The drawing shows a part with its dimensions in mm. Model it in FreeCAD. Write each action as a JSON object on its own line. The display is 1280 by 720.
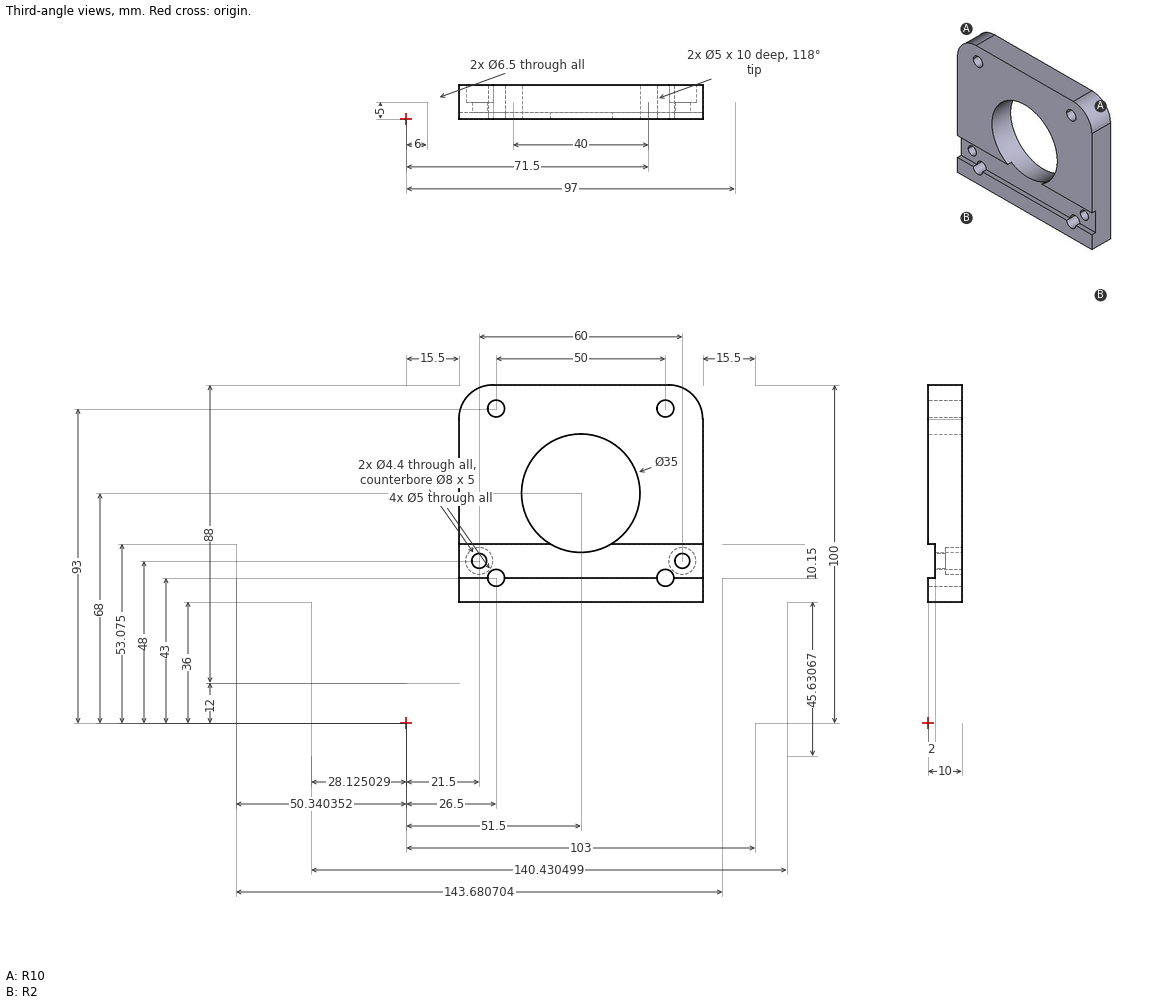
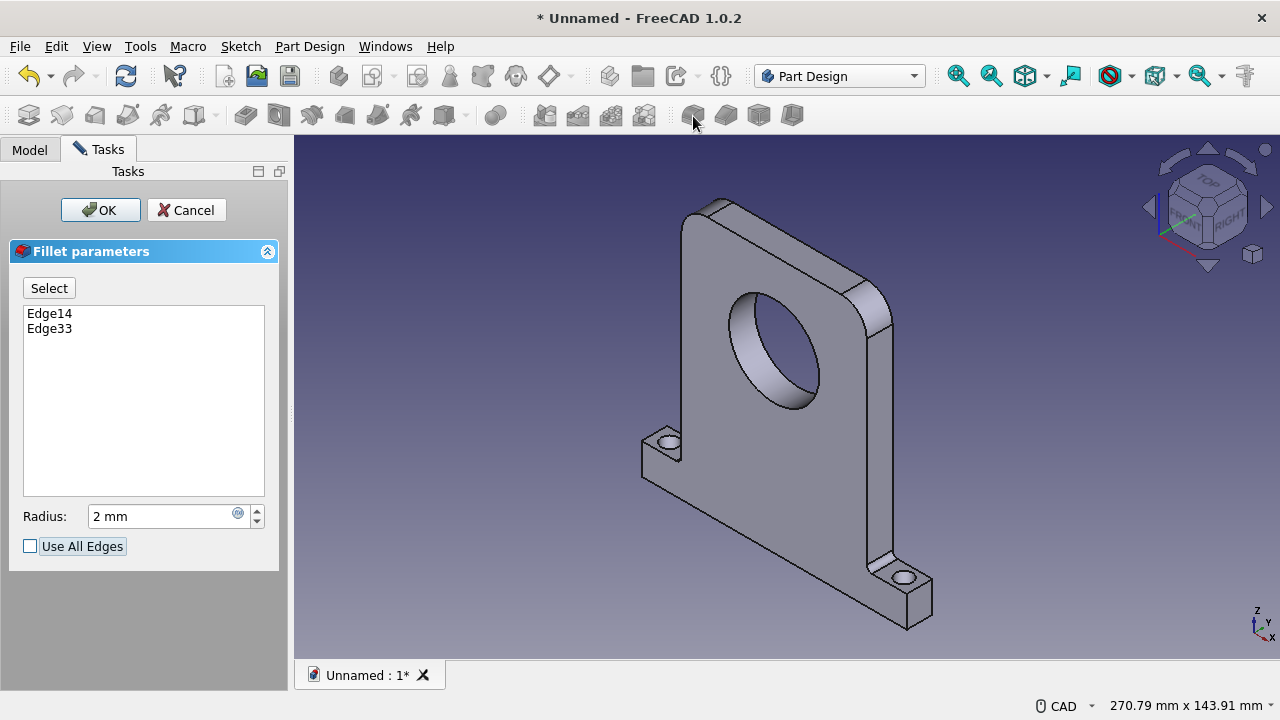
{"action": "left_click", "coordinate": [101, 210]}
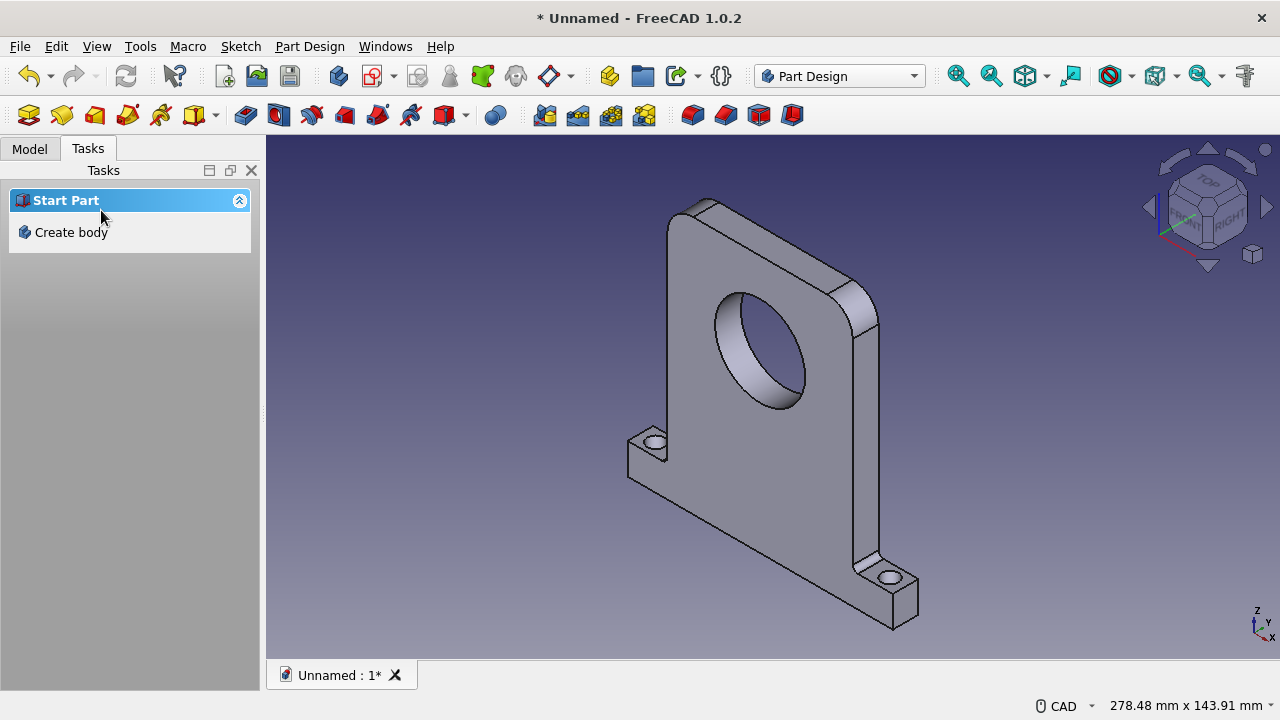
{"action": "key", "text": "4"}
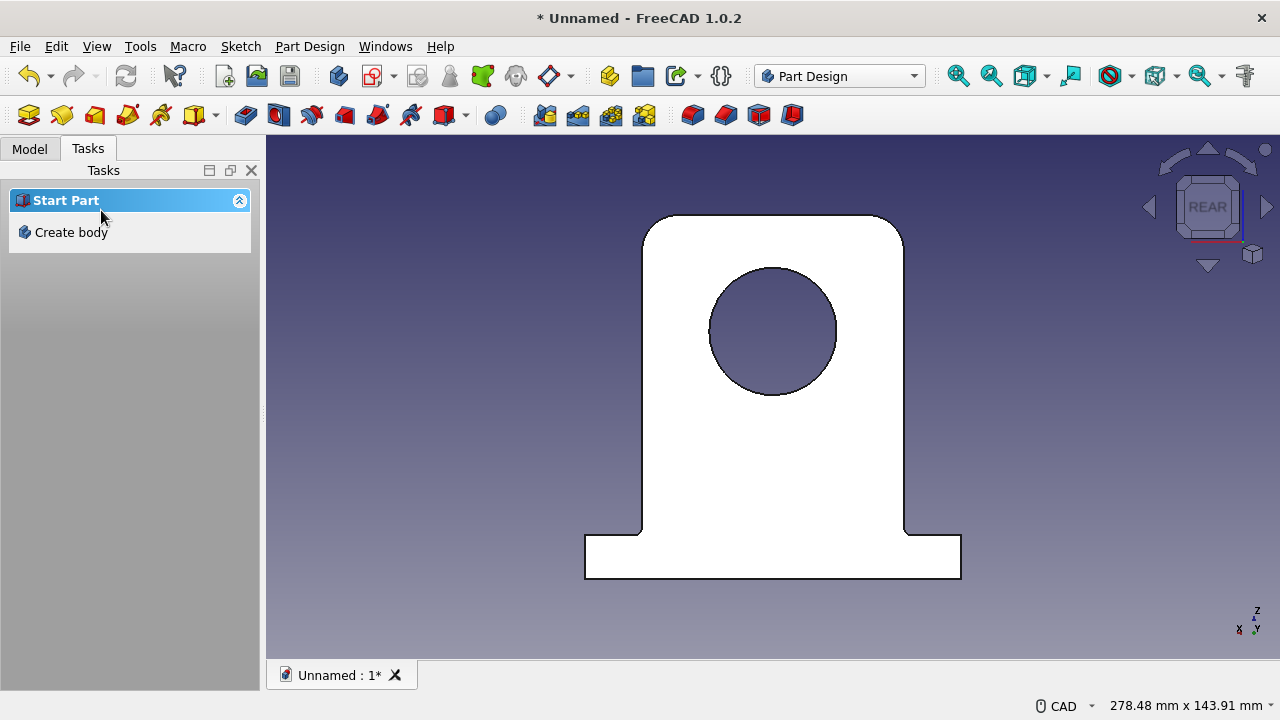
{"action": "left_click", "coordinate": [773, 500]}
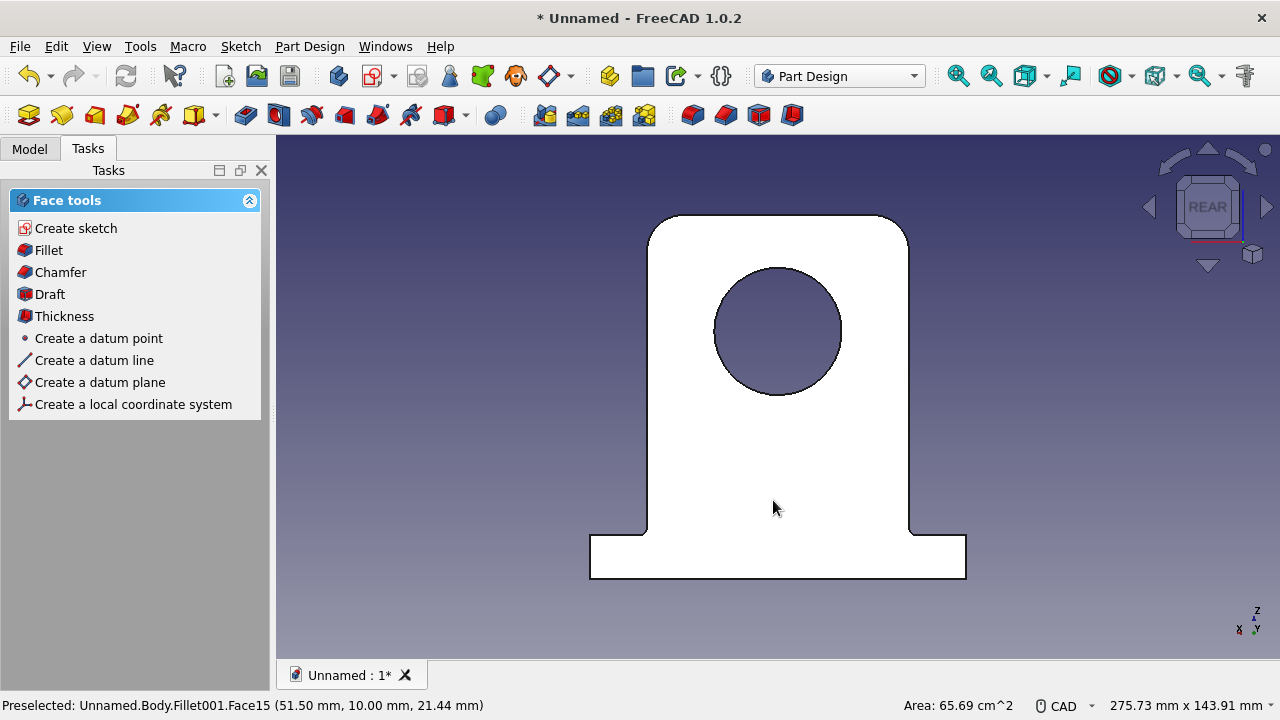
{"action": "left_click", "coordinate": [372, 76]}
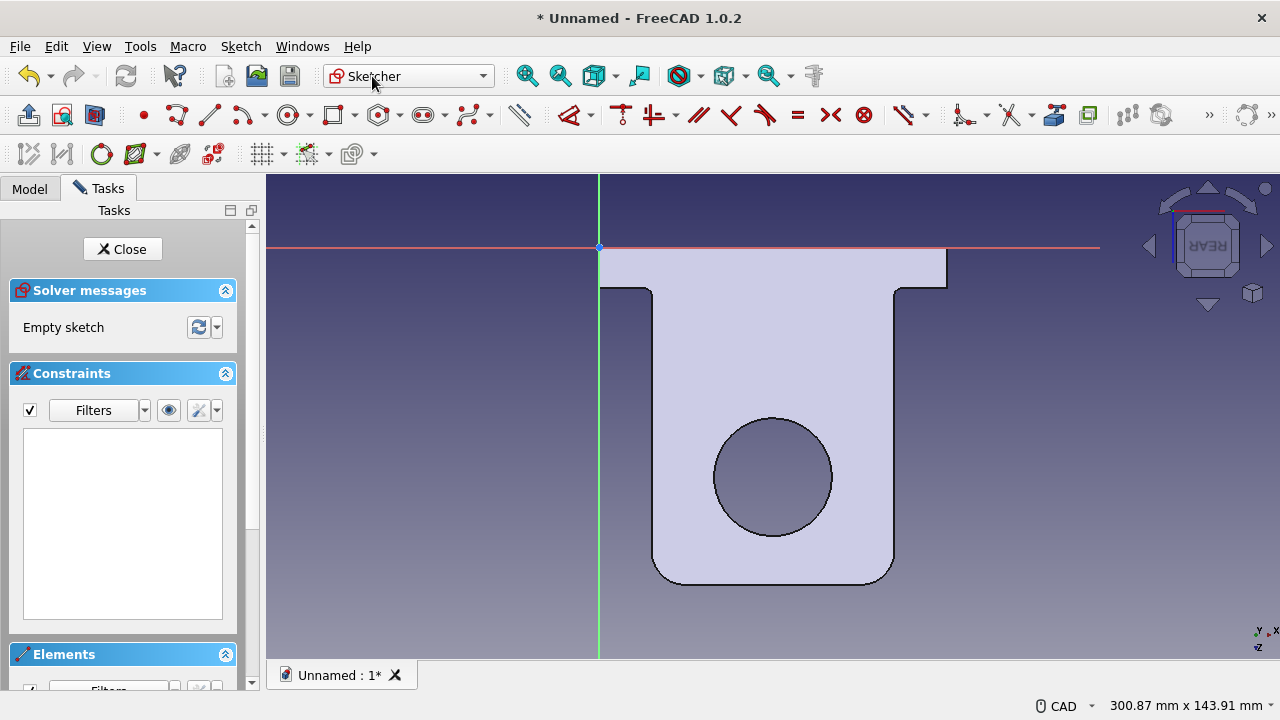
{"action": "scroll", "coordinate": [538, 631], "scroll_direction": "down", "scroll_amount": 1}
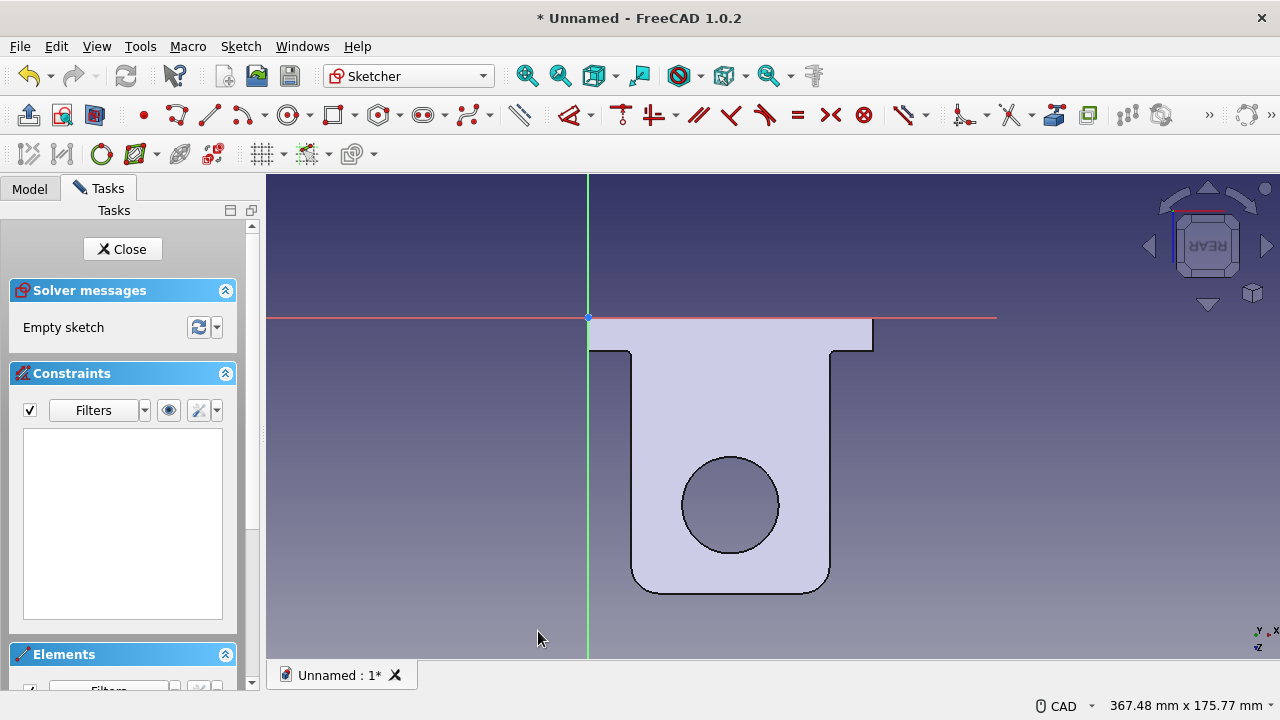
{"action": "scroll", "coordinate": [704, 227], "scroll_direction": "up", "scroll_amount": 2}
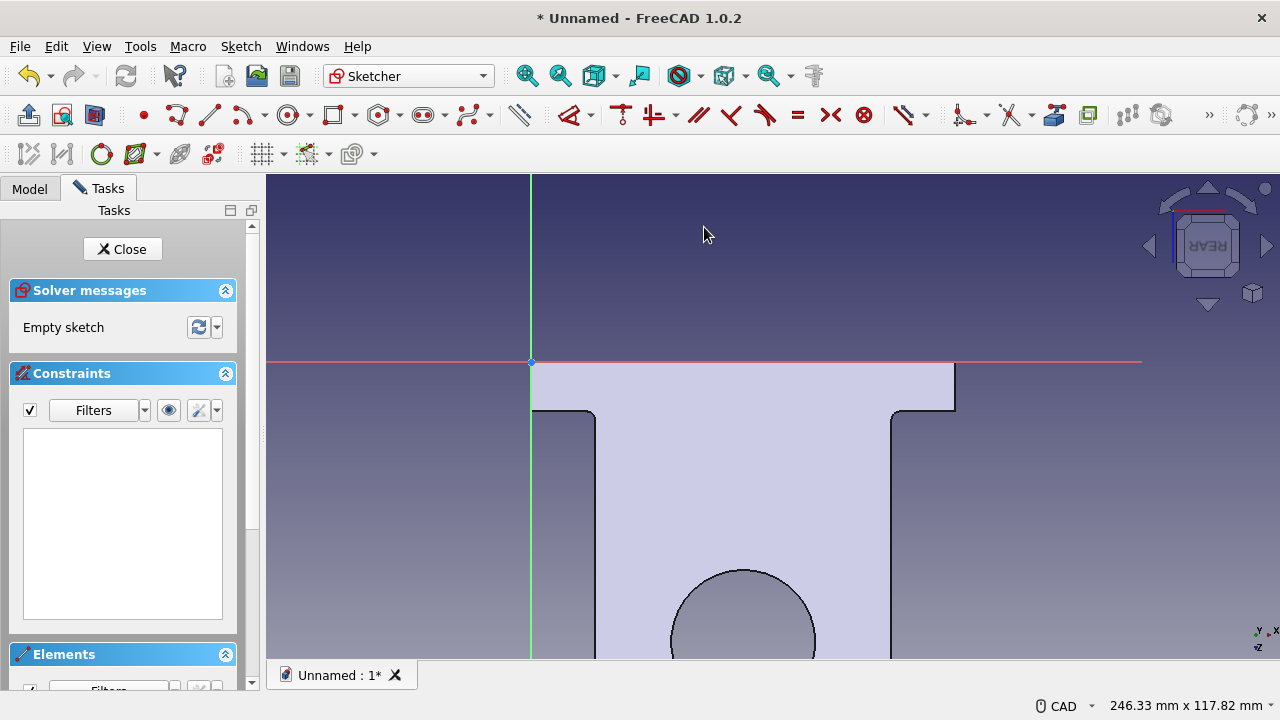
{"action": "left_click", "coordinate": [332, 116]}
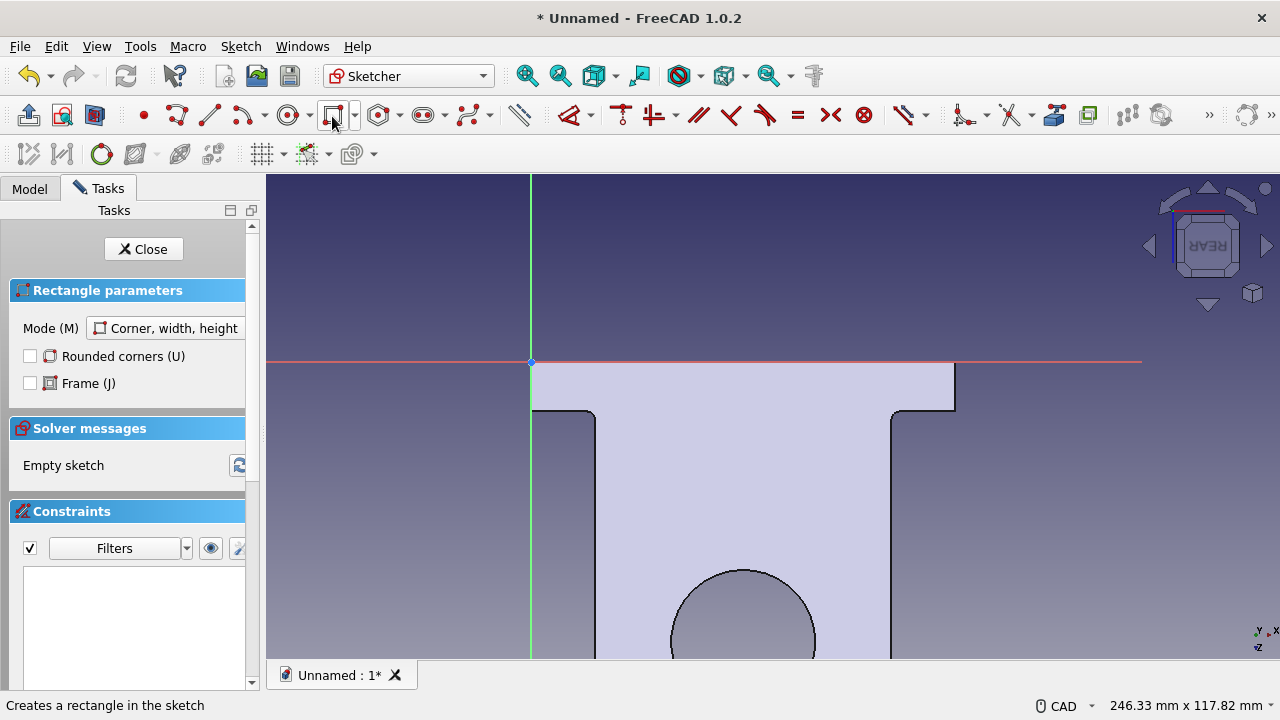
{"action": "left_click", "coordinate": [415, 322]}
{"action": "mouse_move", "coordinate": [994, 510]}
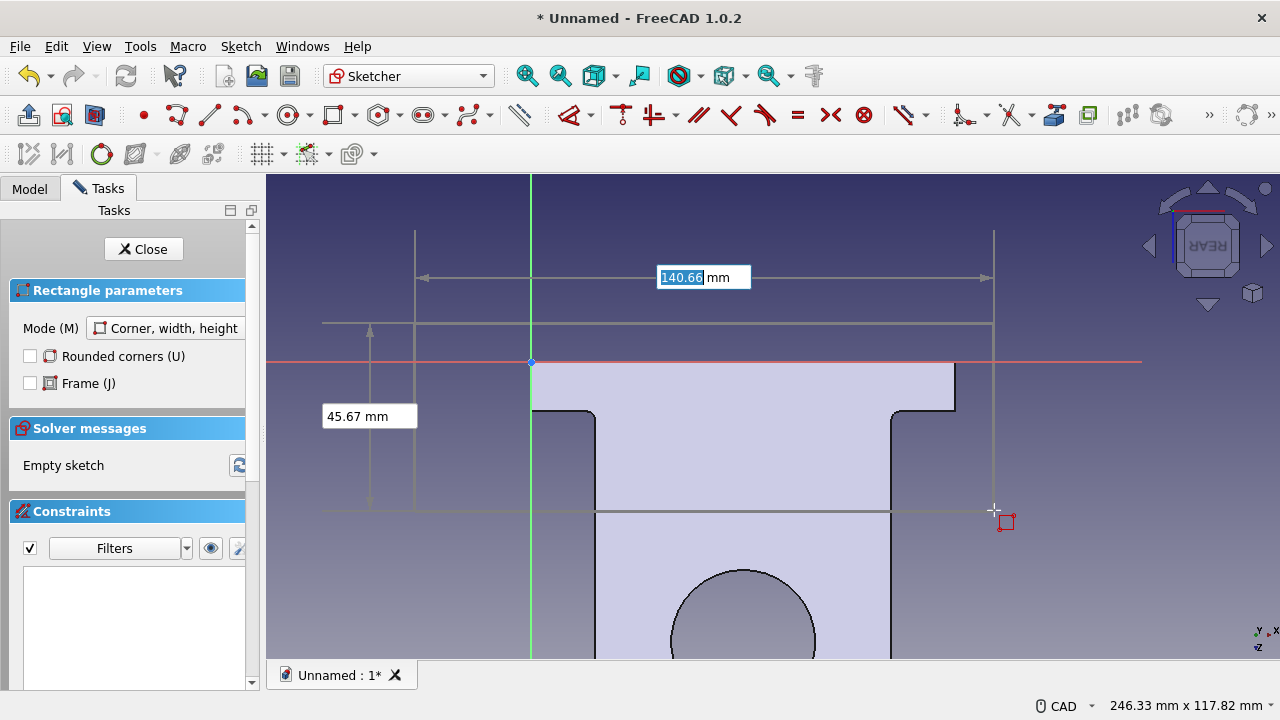
{"action": "type", "text": "140.430499"}
{"action": "key", "text": "Tab"}
{"action": "type", "text": "45.63067"}
{"action": "key", "text": "Return"}
{"action": "key", "text": "Escape"}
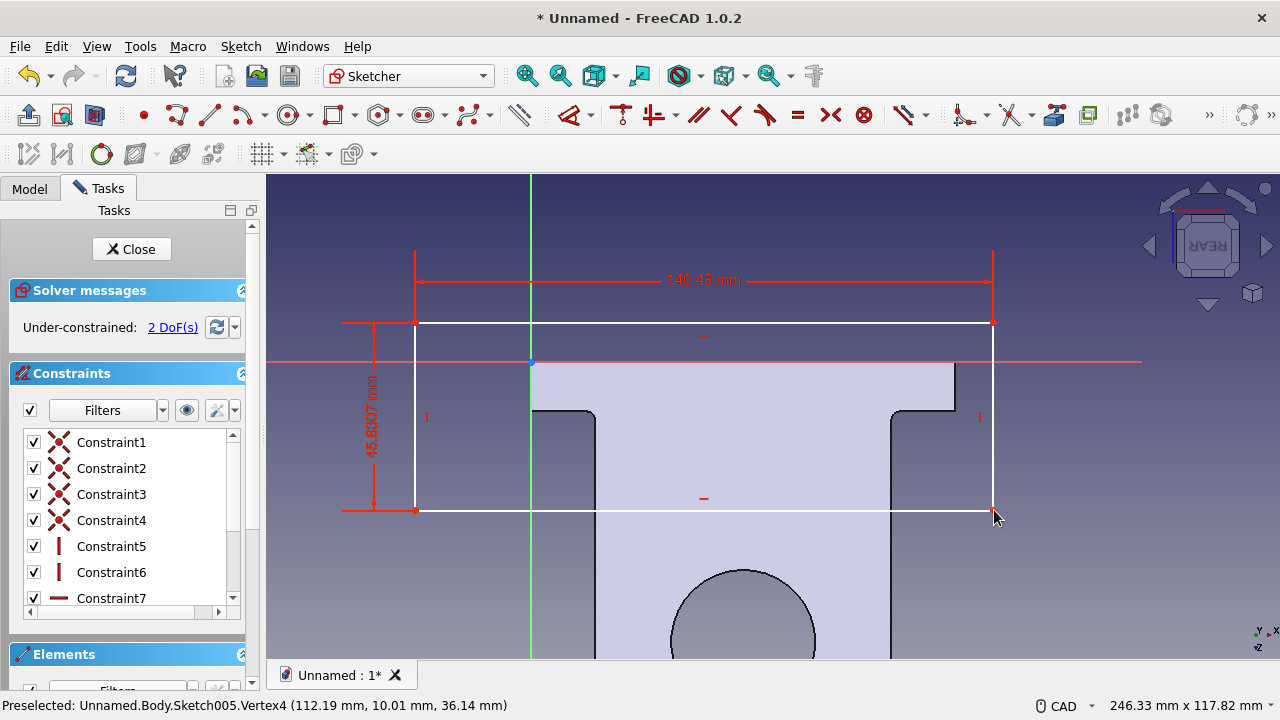
{"action": "left_click", "coordinate": [568, 116]}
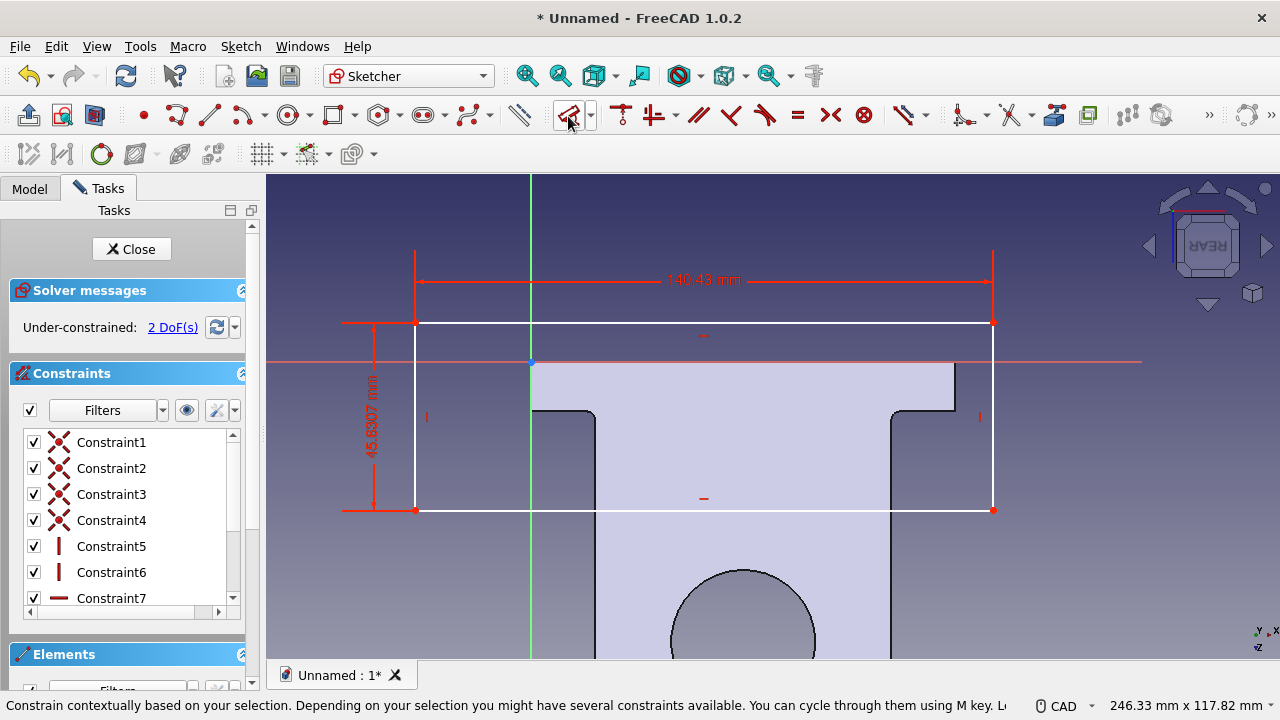
{"action": "left_click", "coordinate": [415, 511]}
{"action": "left_click", "coordinate": [381, 436]}